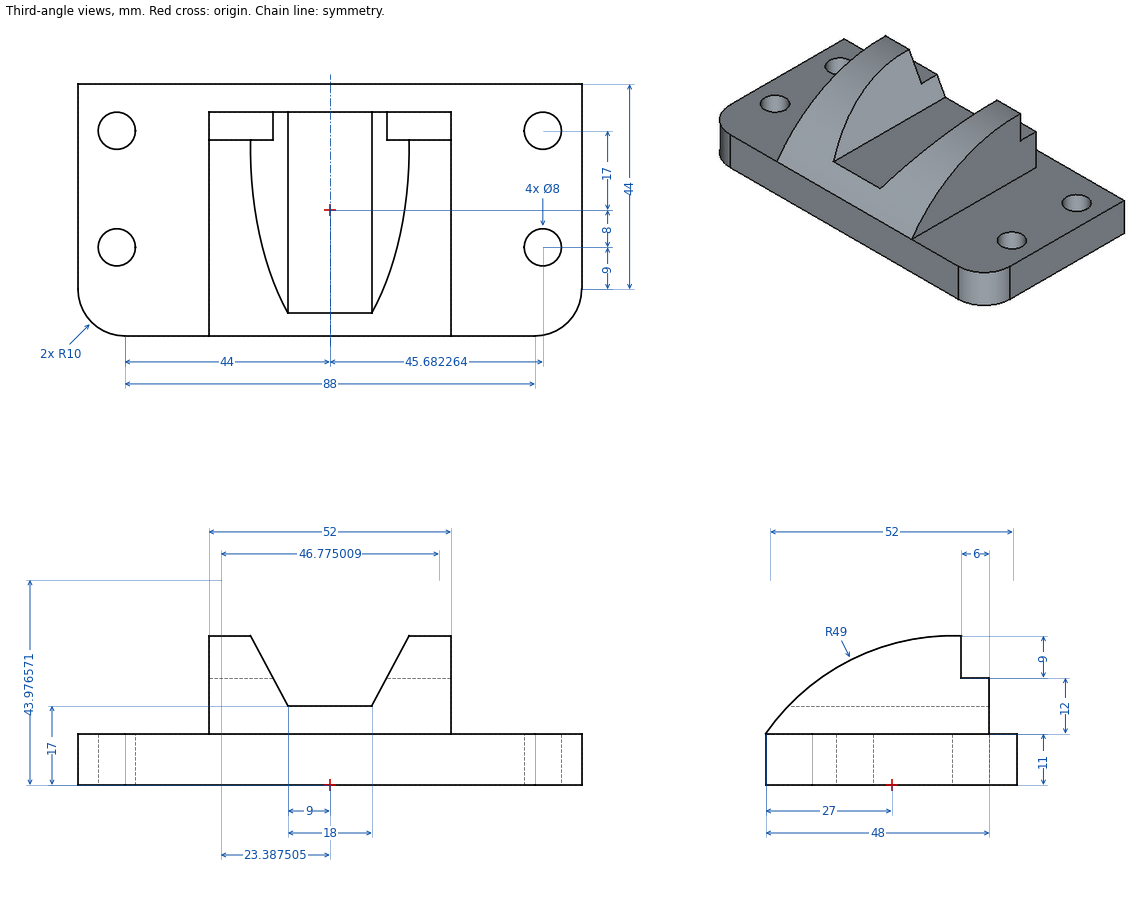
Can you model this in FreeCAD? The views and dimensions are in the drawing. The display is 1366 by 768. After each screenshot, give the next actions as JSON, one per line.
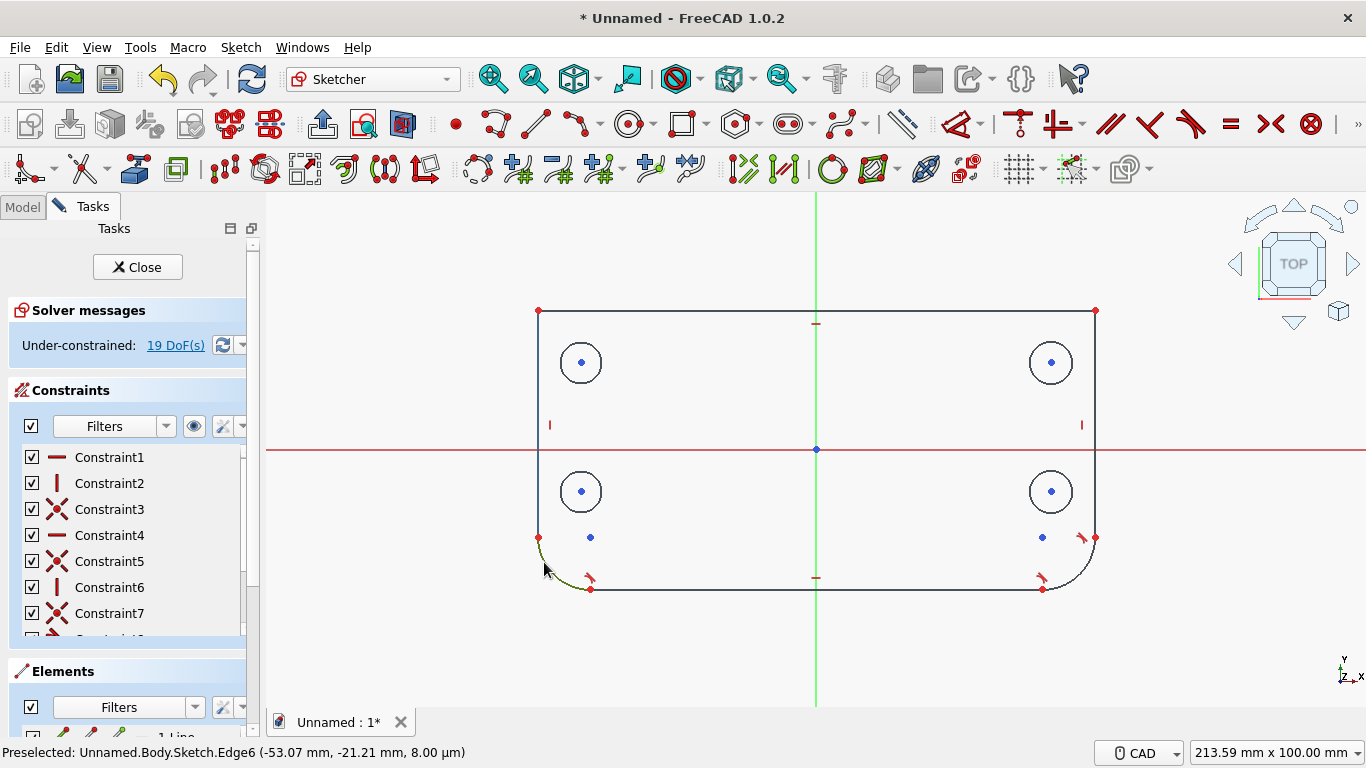
{"action": "key", "text": "t"}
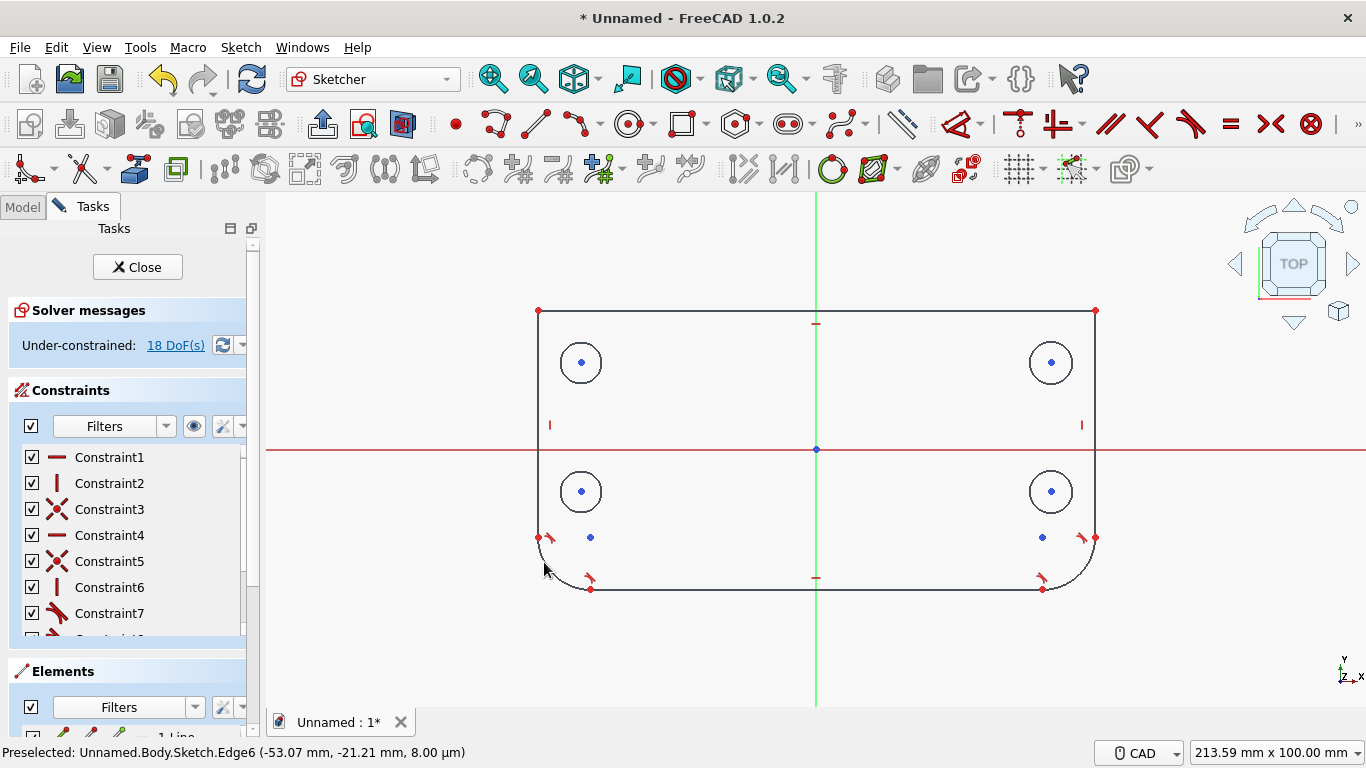
{"action": "left_click", "coordinate": [1066, 584]}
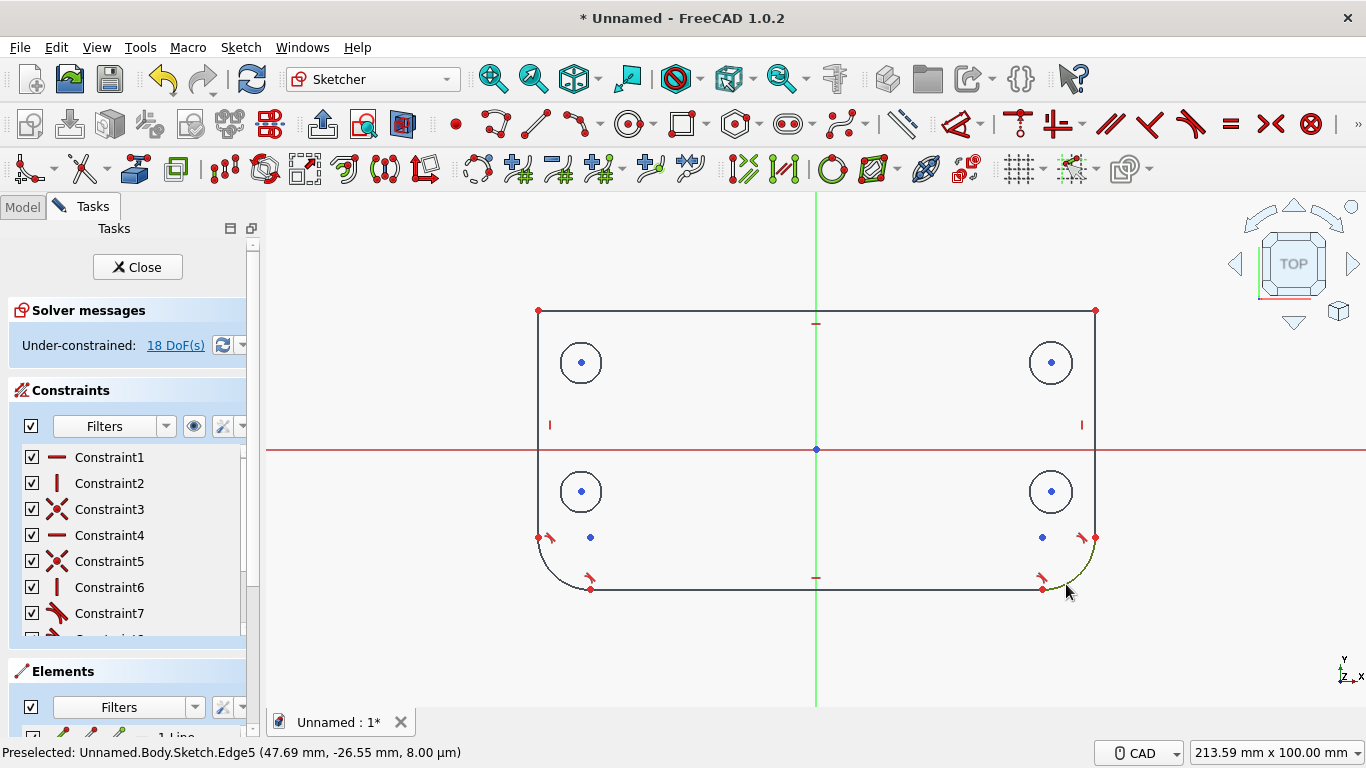
{"action": "left_click", "coordinate": [544, 561]}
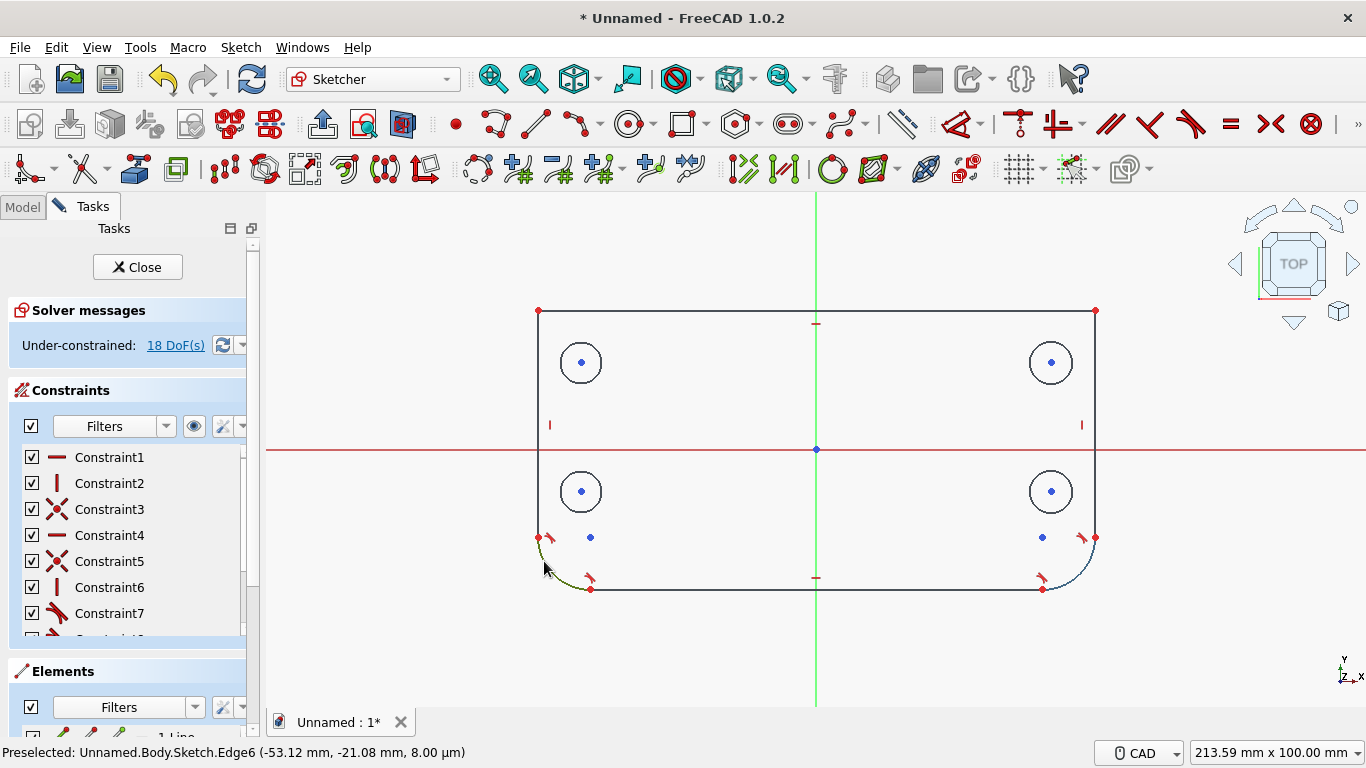
{"action": "key", "text": "e"}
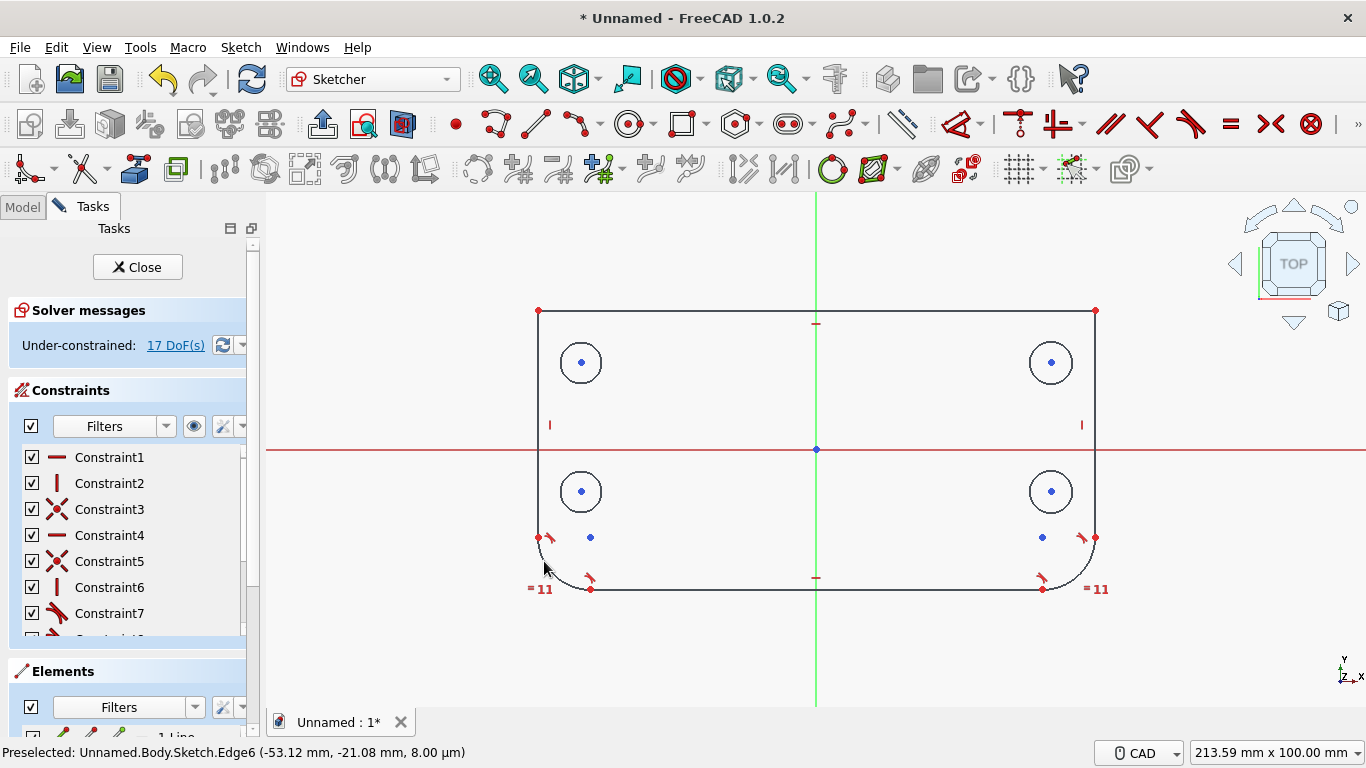
{"action": "left_click", "coordinate": [1066, 477]}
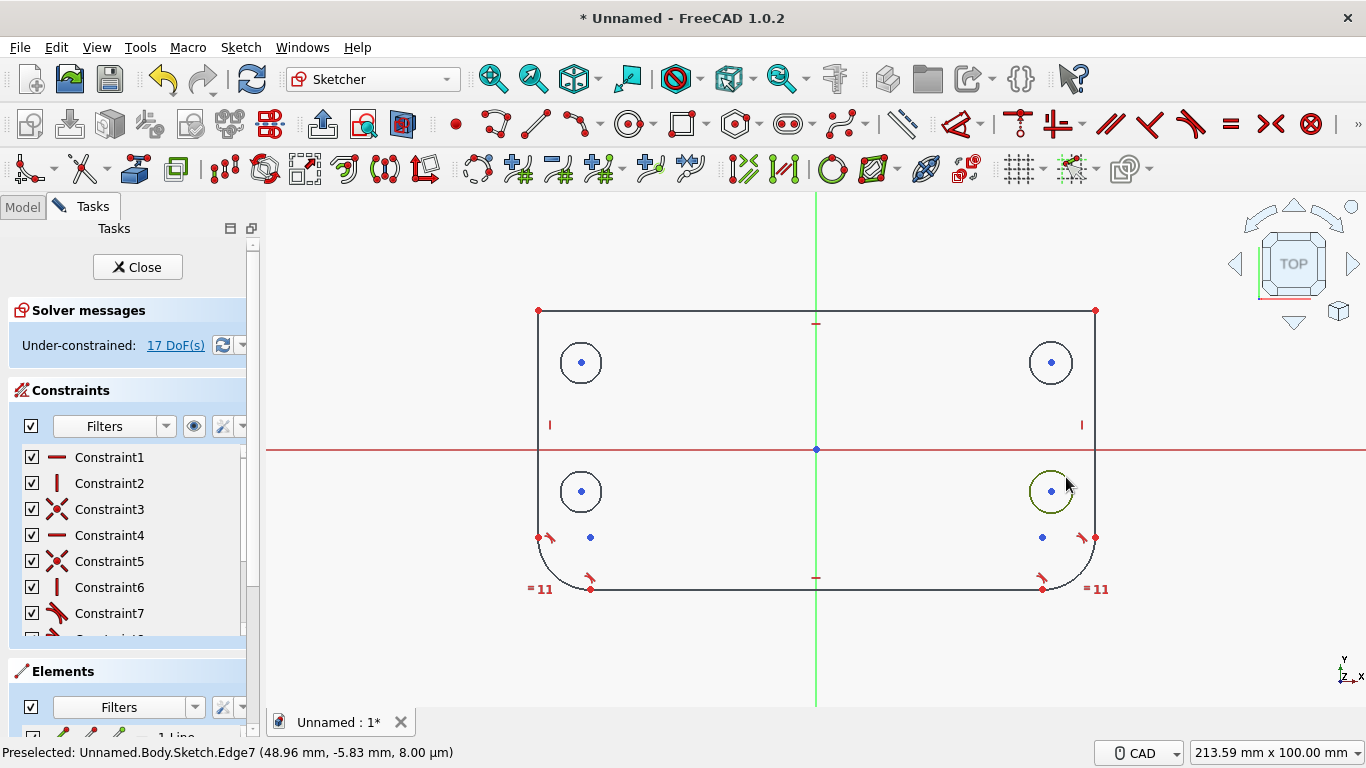
{"action": "left_click", "coordinate": [595, 477]}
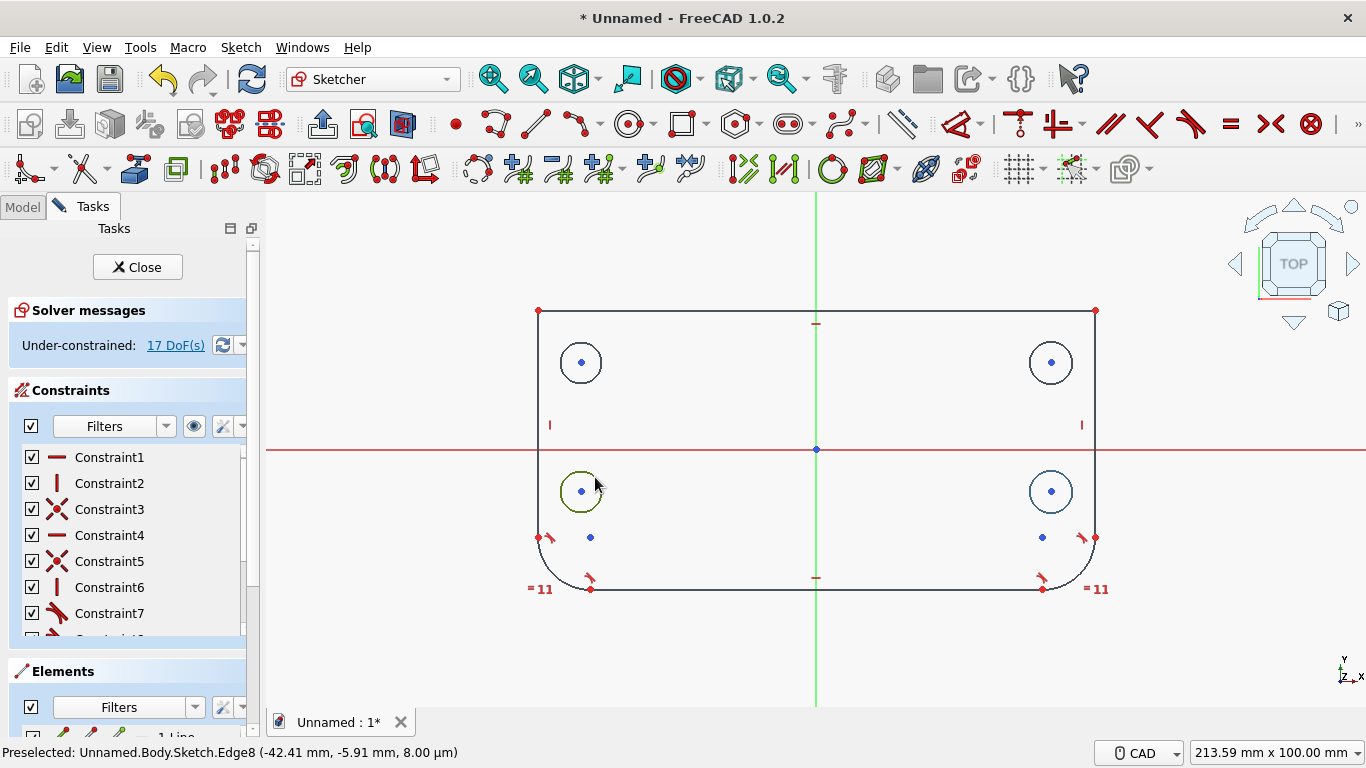
{"action": "left_click", "coordinate": [1066, 348]}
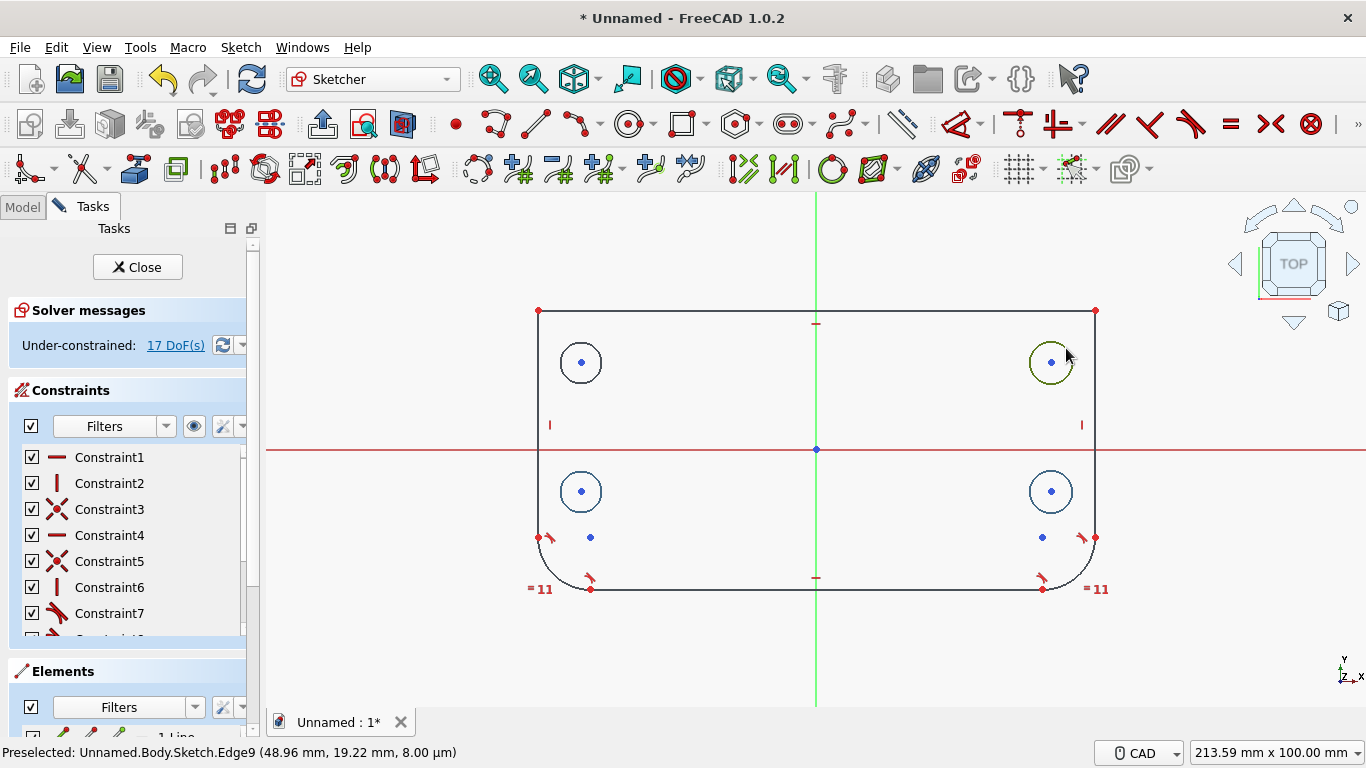
{"action": "left_click", "coordinate": [595, 348]}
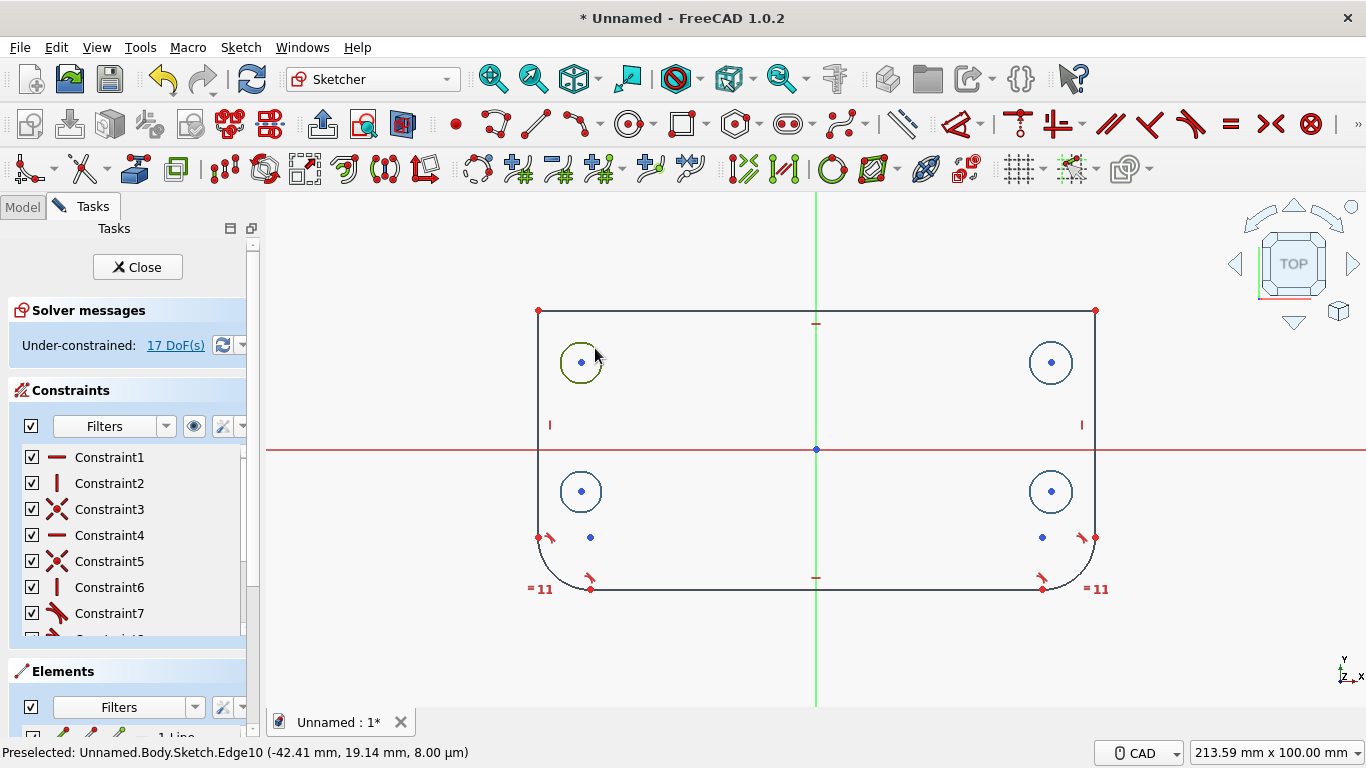
{"action": "key", "text": "e"}